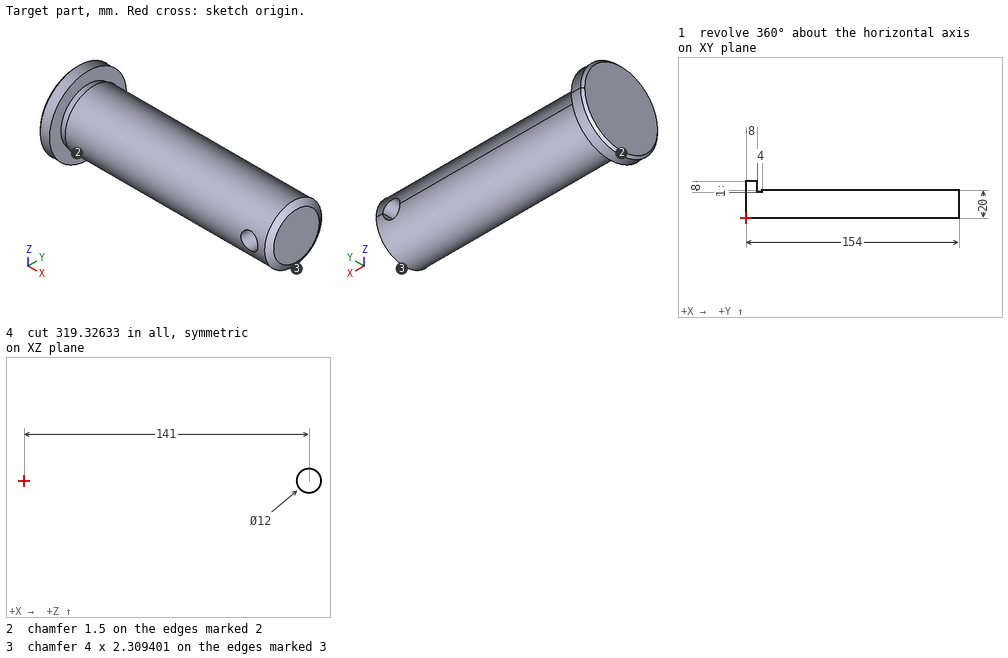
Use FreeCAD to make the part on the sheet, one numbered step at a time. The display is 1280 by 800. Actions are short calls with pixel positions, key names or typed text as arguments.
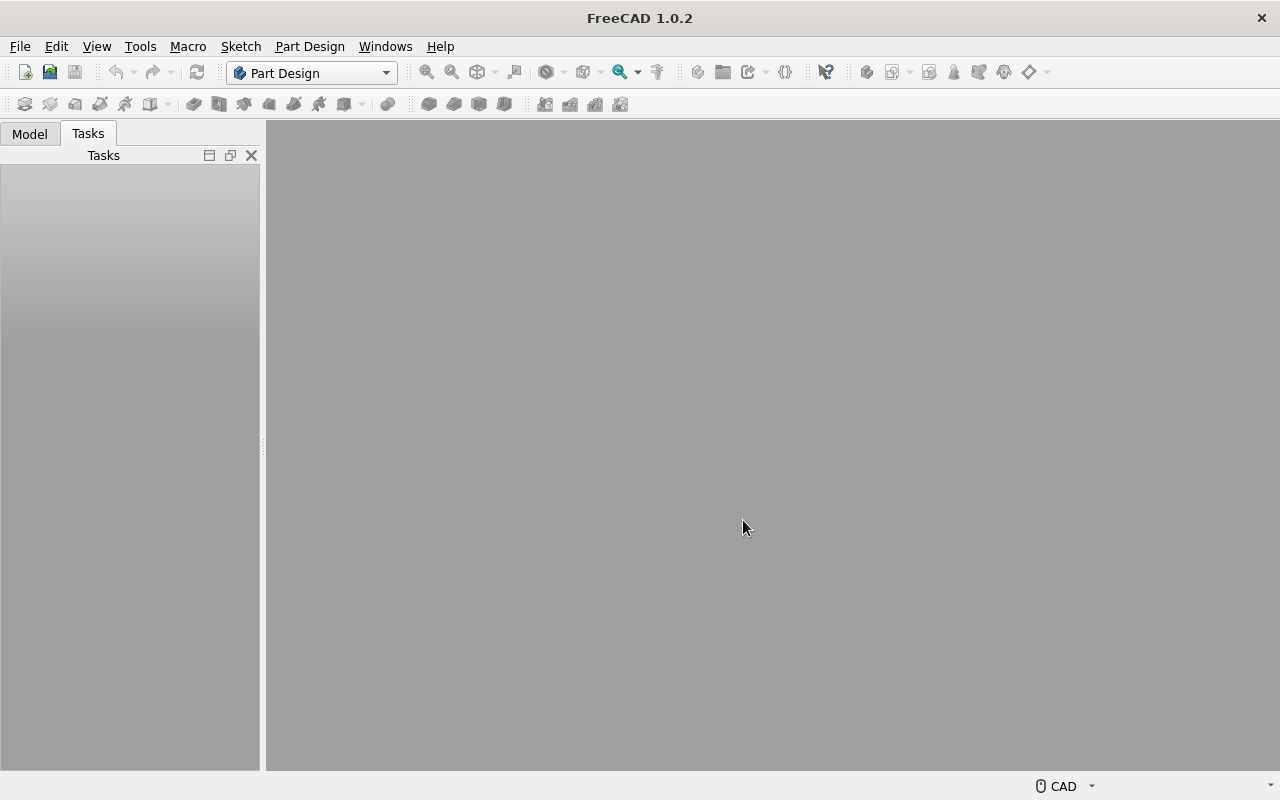
click(25, 72)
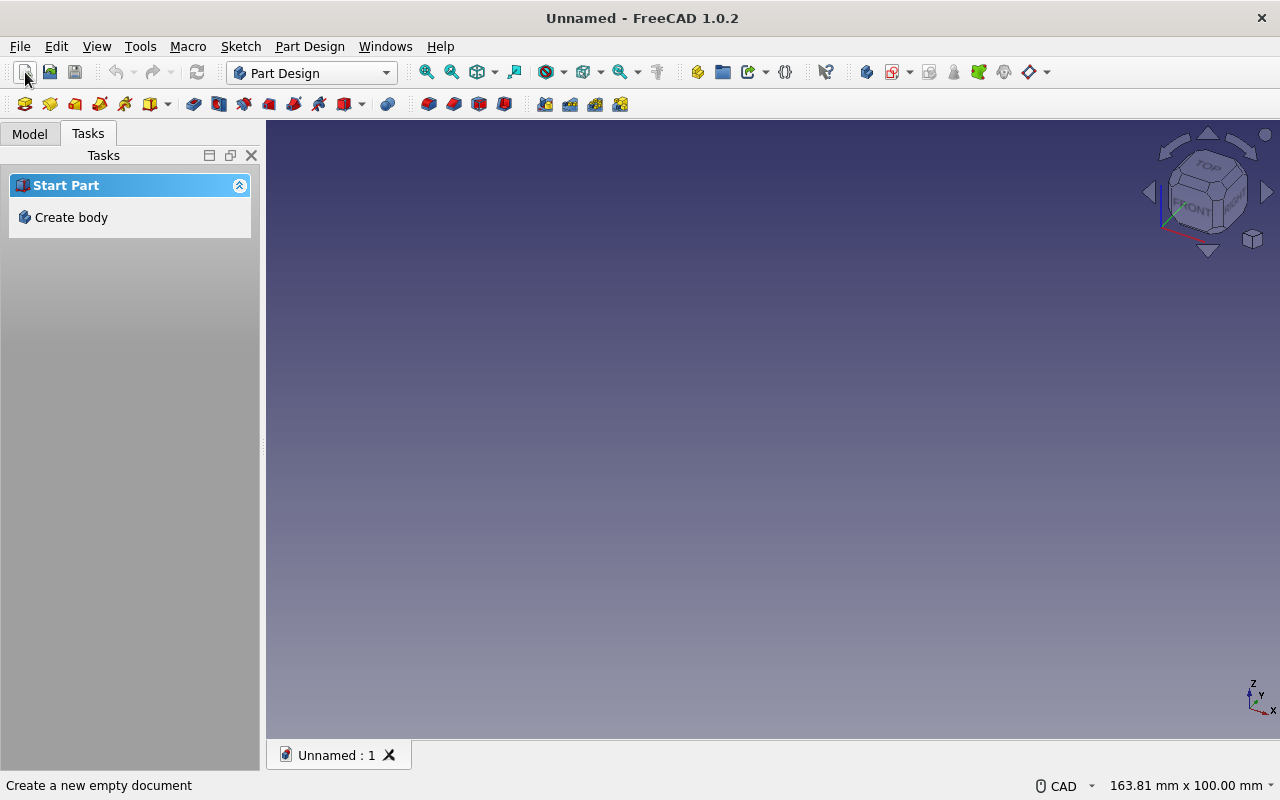
click(892, 72)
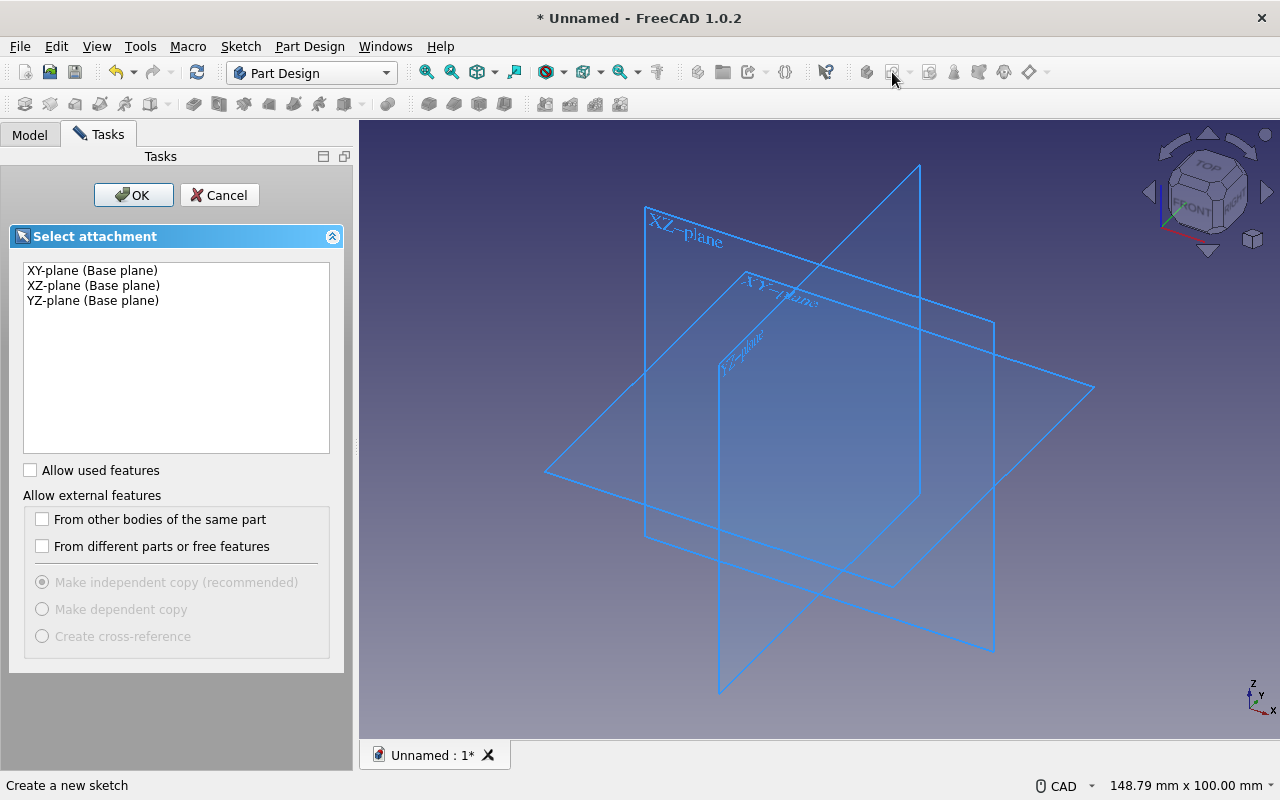
click(84, 270)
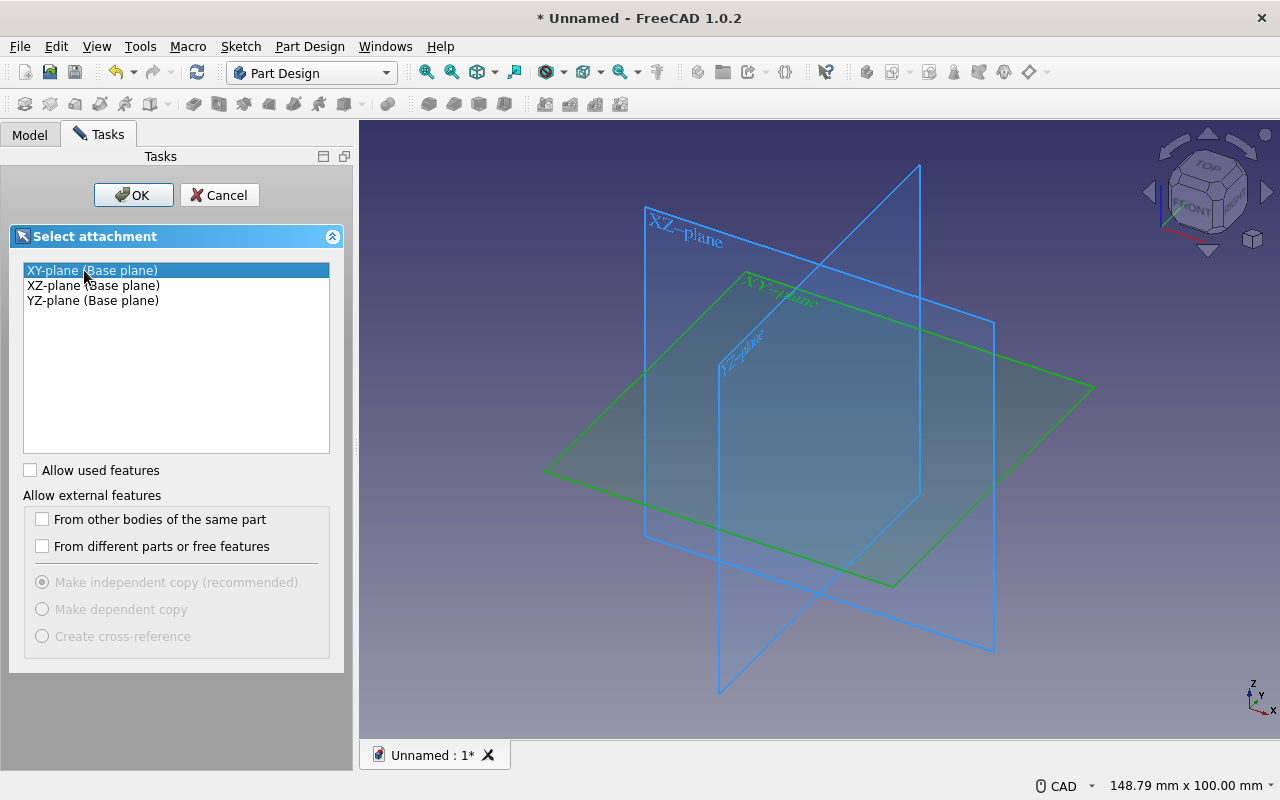
click(134, 195)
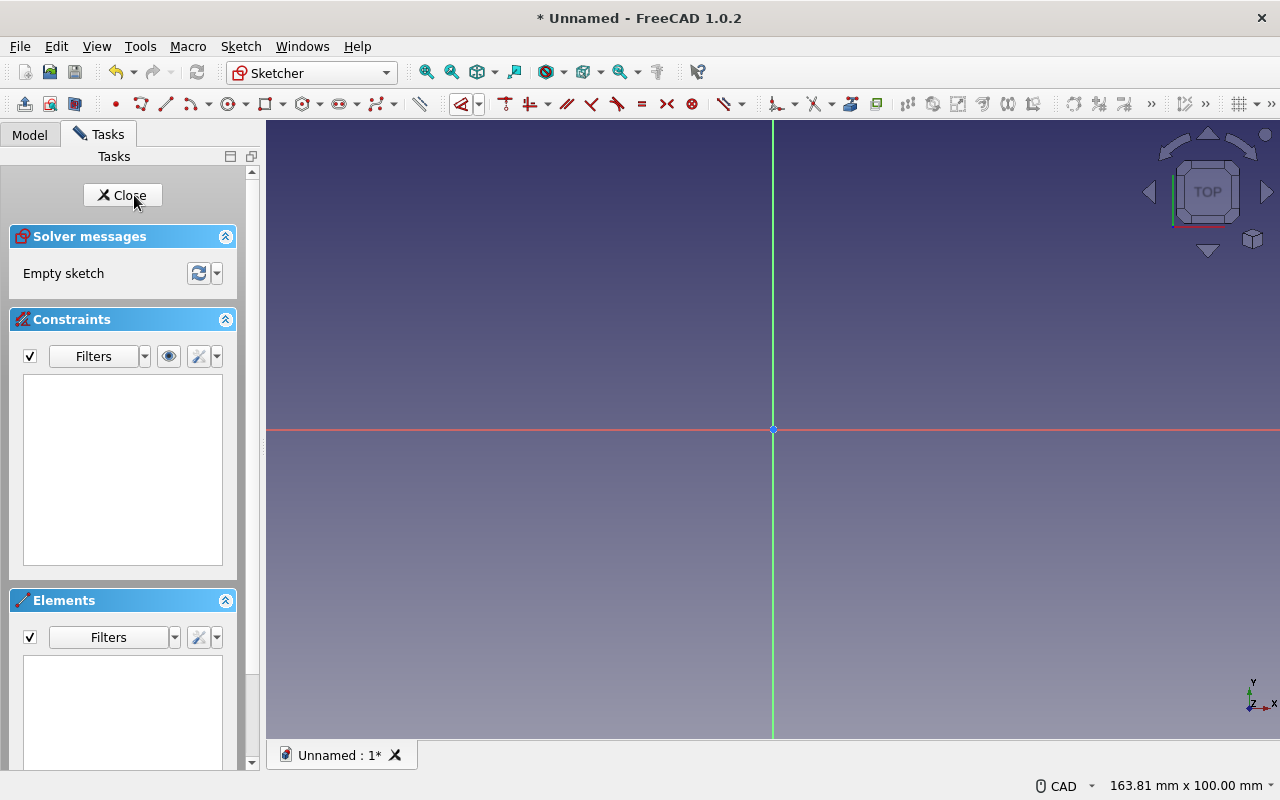
scroll(294, 531, down, 3)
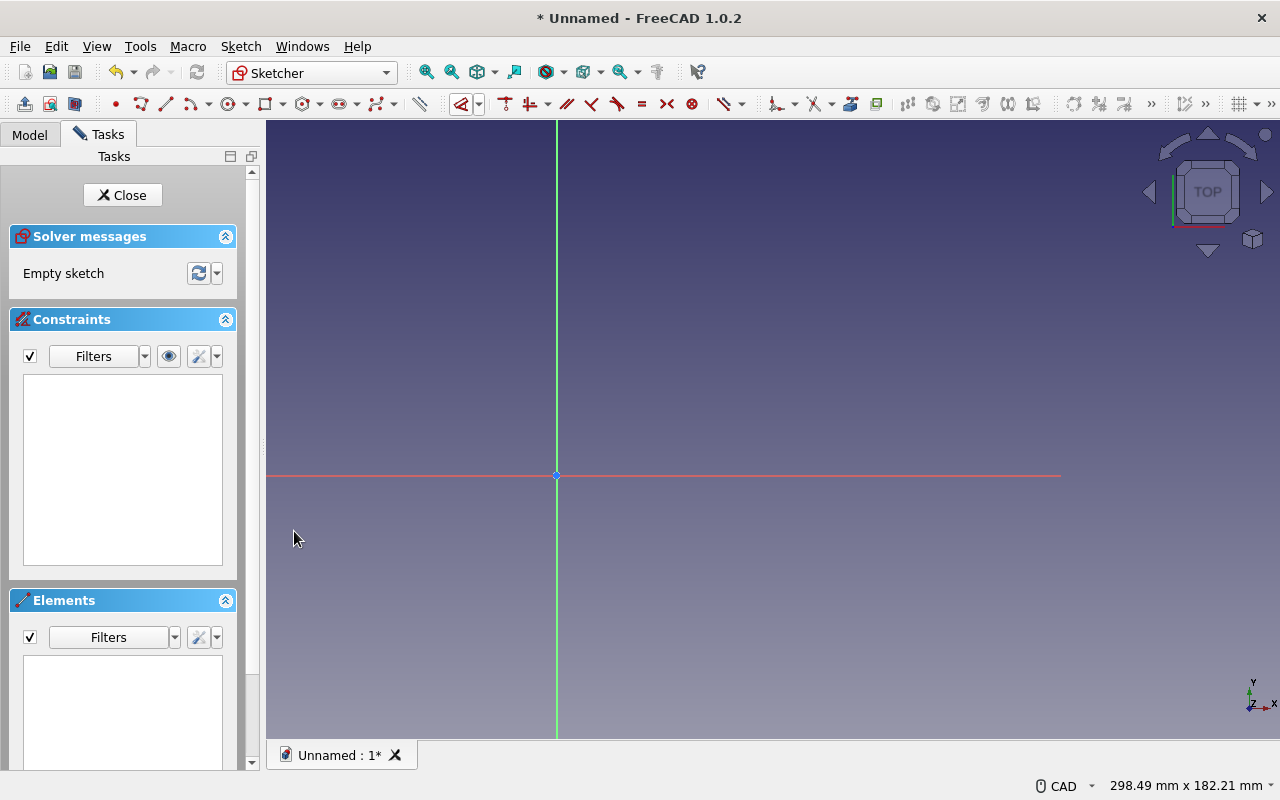
click(141, 104)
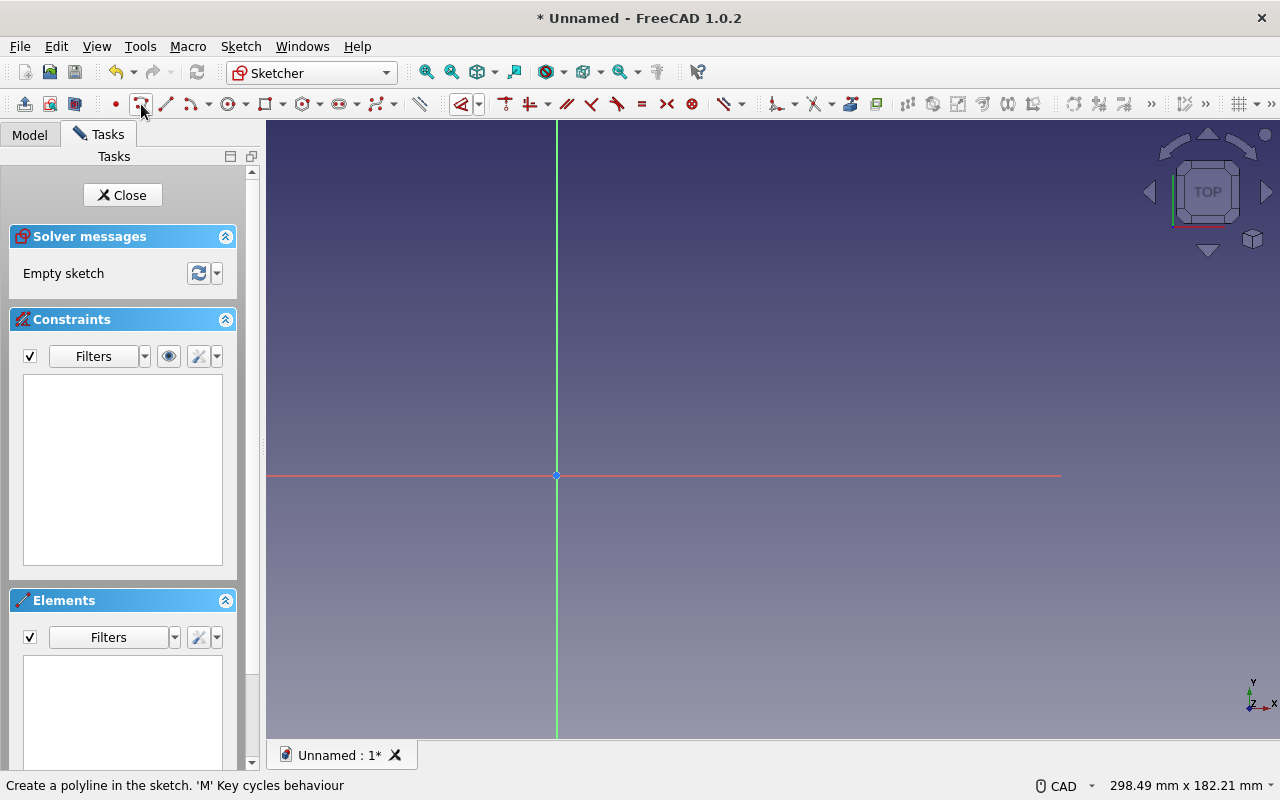
click(557, 476)
click(1080, 467)
click(1080, 408)
click(598, 408)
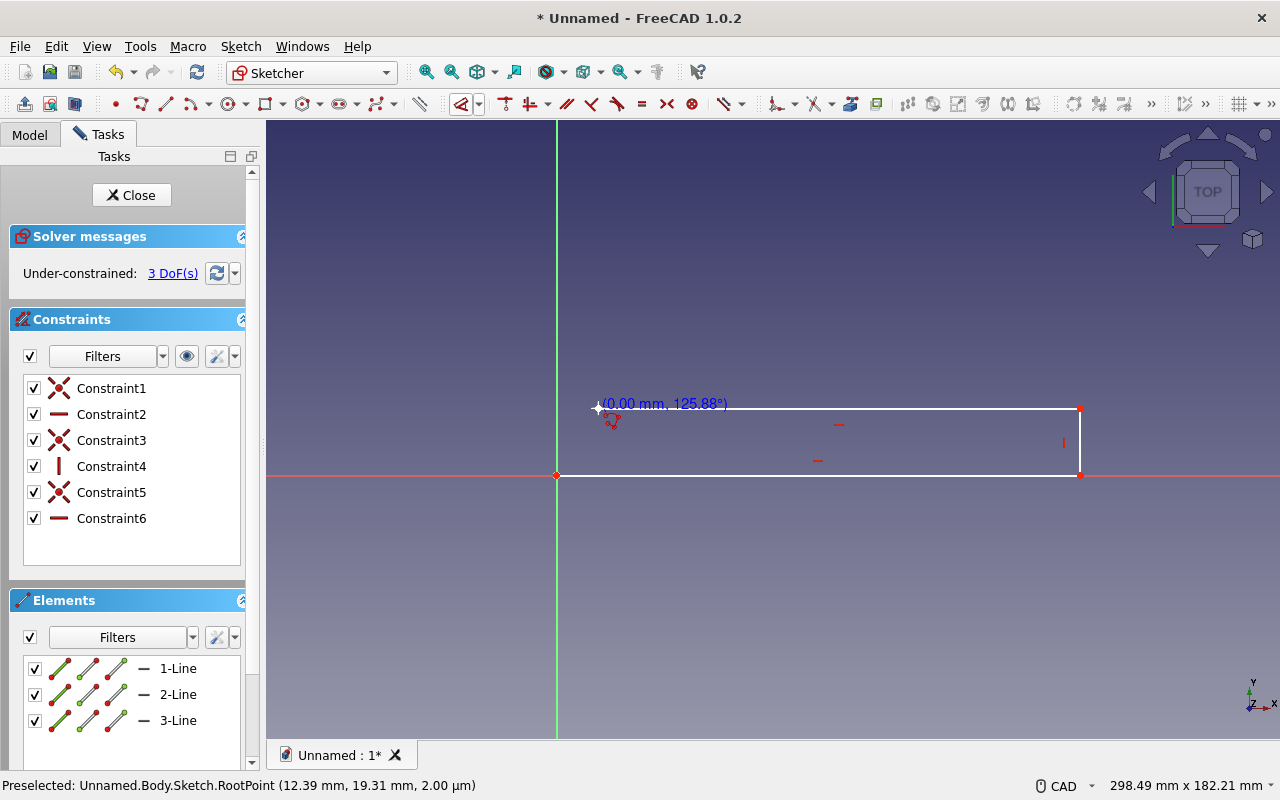
scroll(598, 411, up, 8)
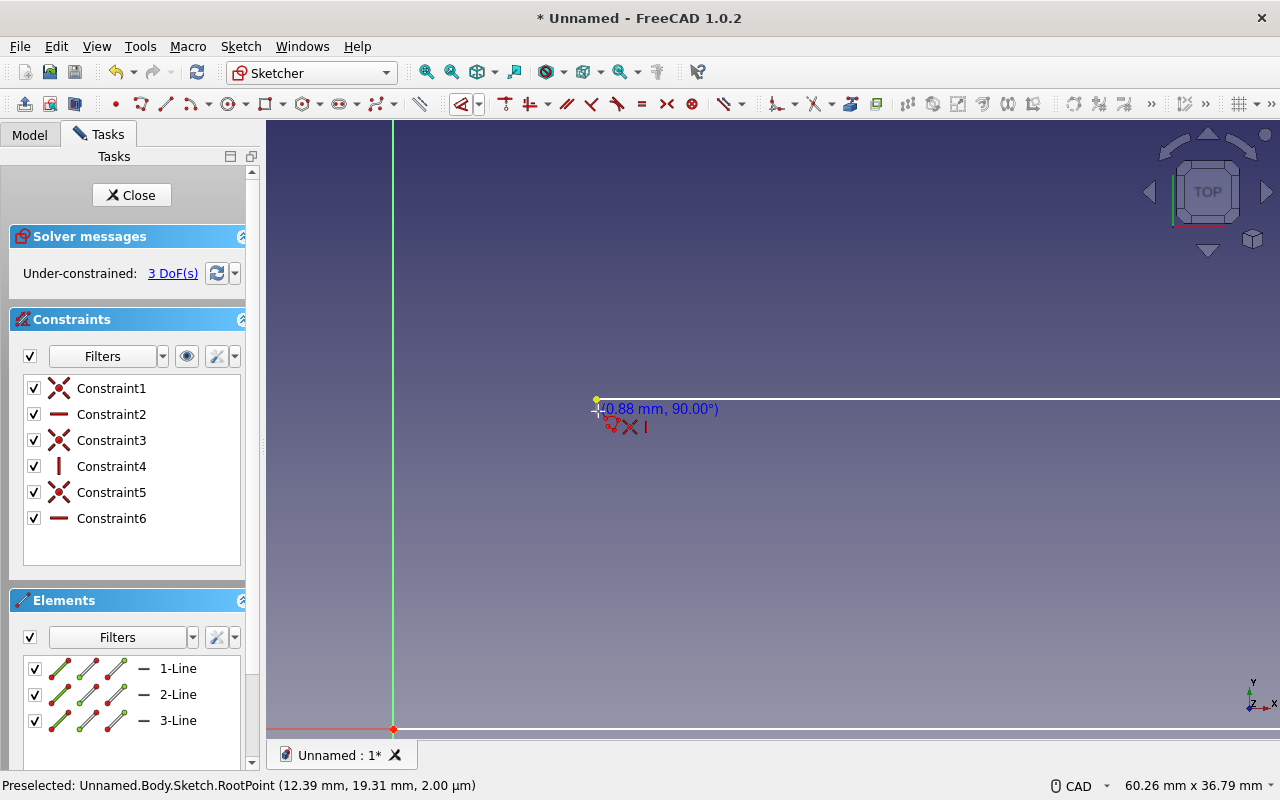
click(597, 409)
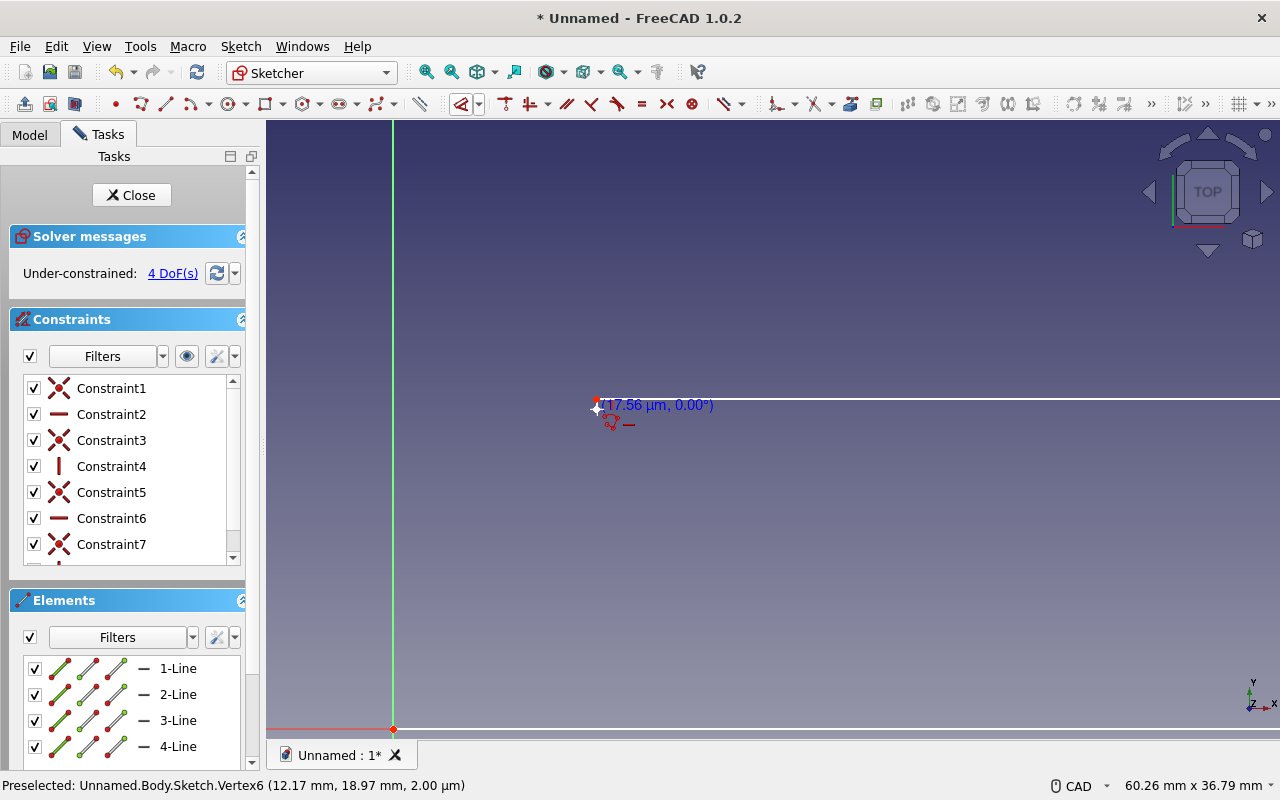
scroll(382, 406, down, 7)